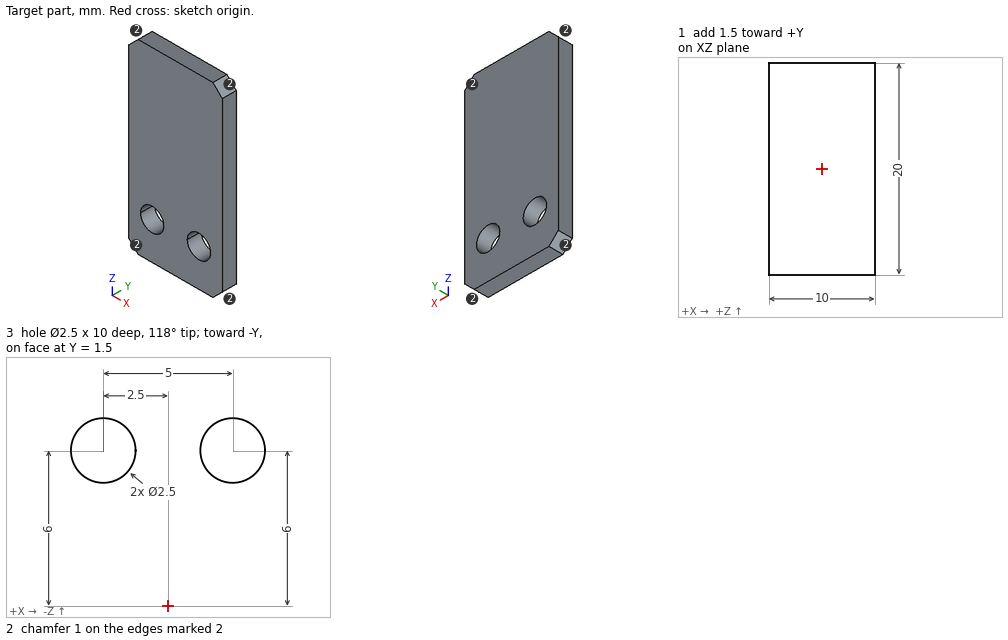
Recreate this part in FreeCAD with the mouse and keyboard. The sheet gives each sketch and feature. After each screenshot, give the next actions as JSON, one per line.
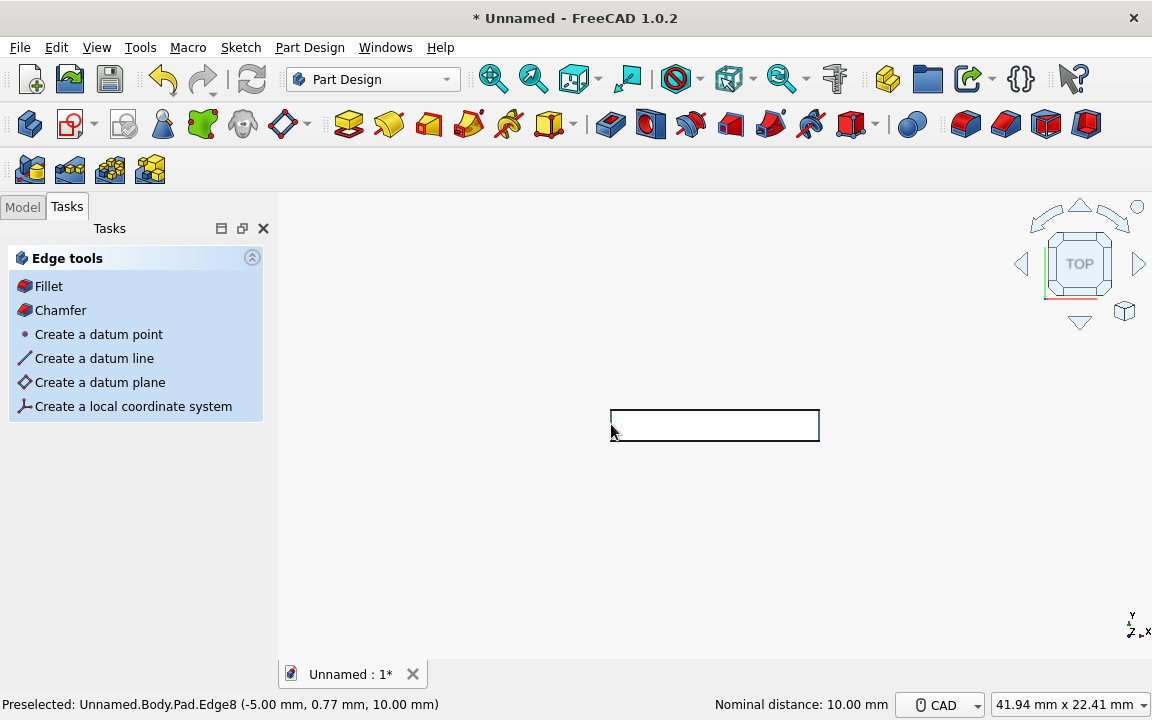
{"action": "key", "text": "1"}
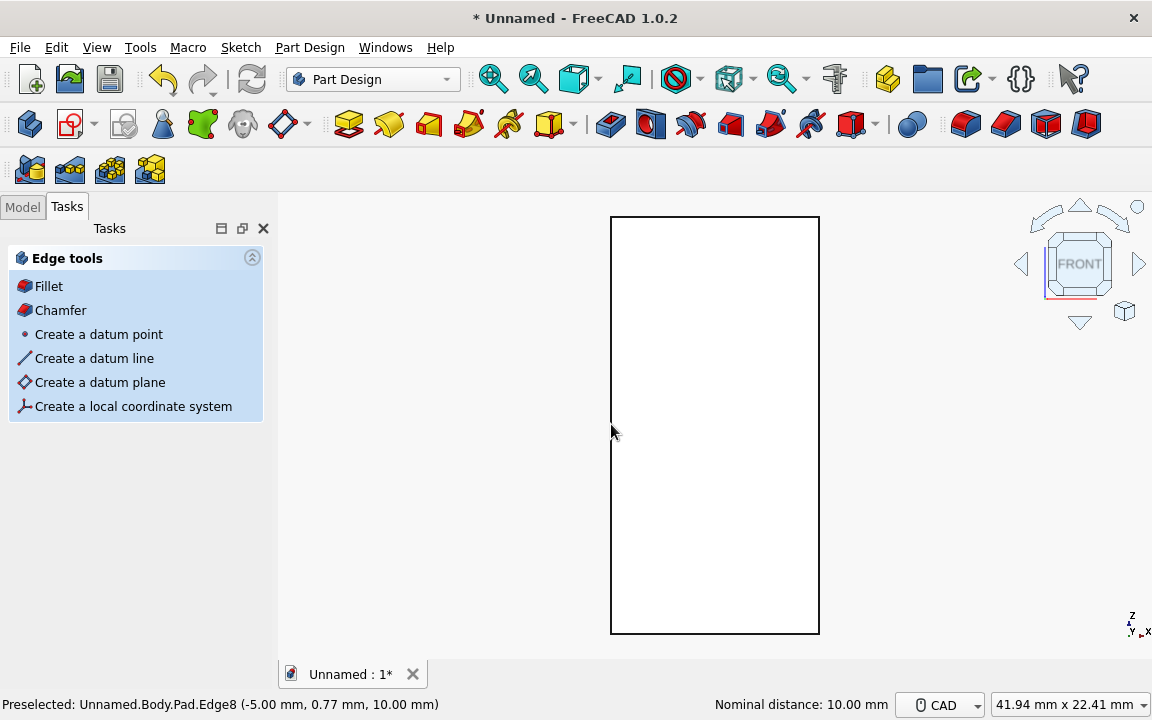
{"action": "key", "text": "3"}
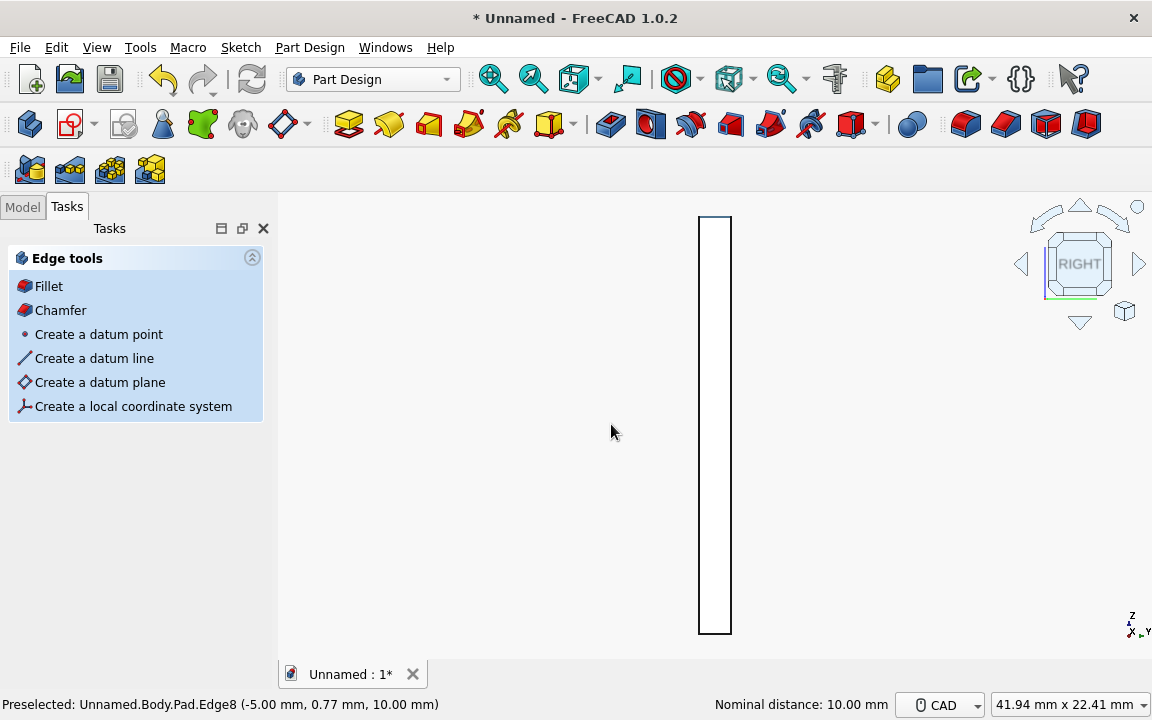
{"action": "key", "text": "5"}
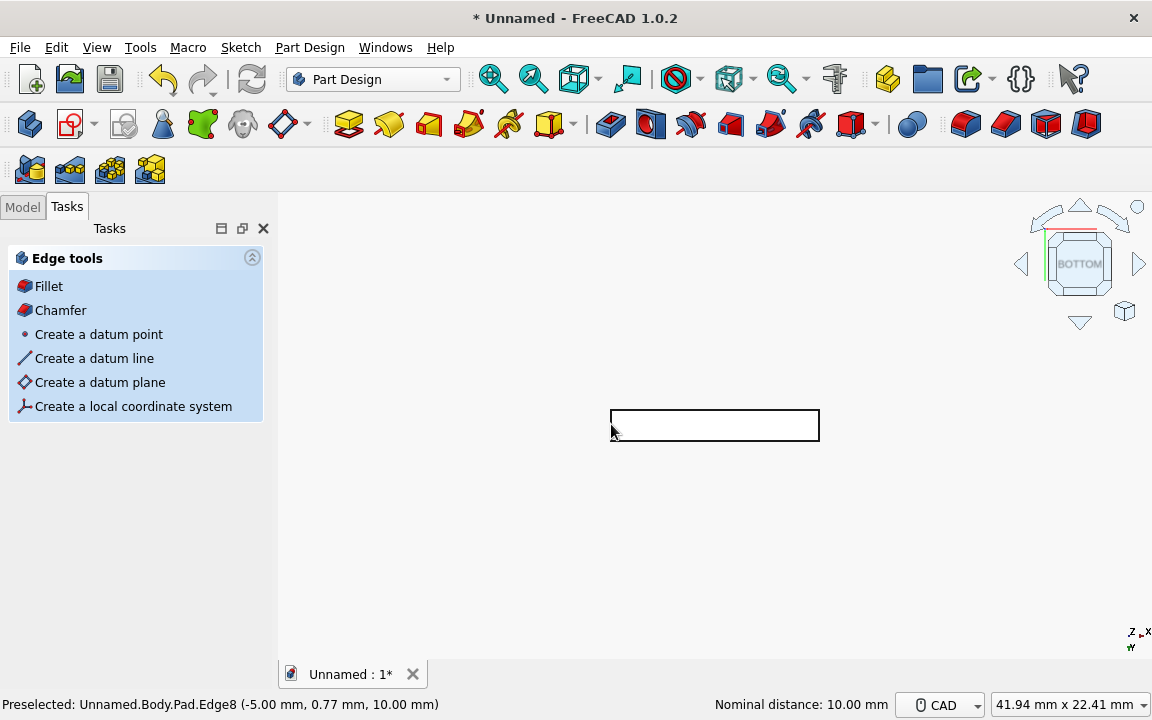
{"action": "left_click", "coordinate": [494, 80]}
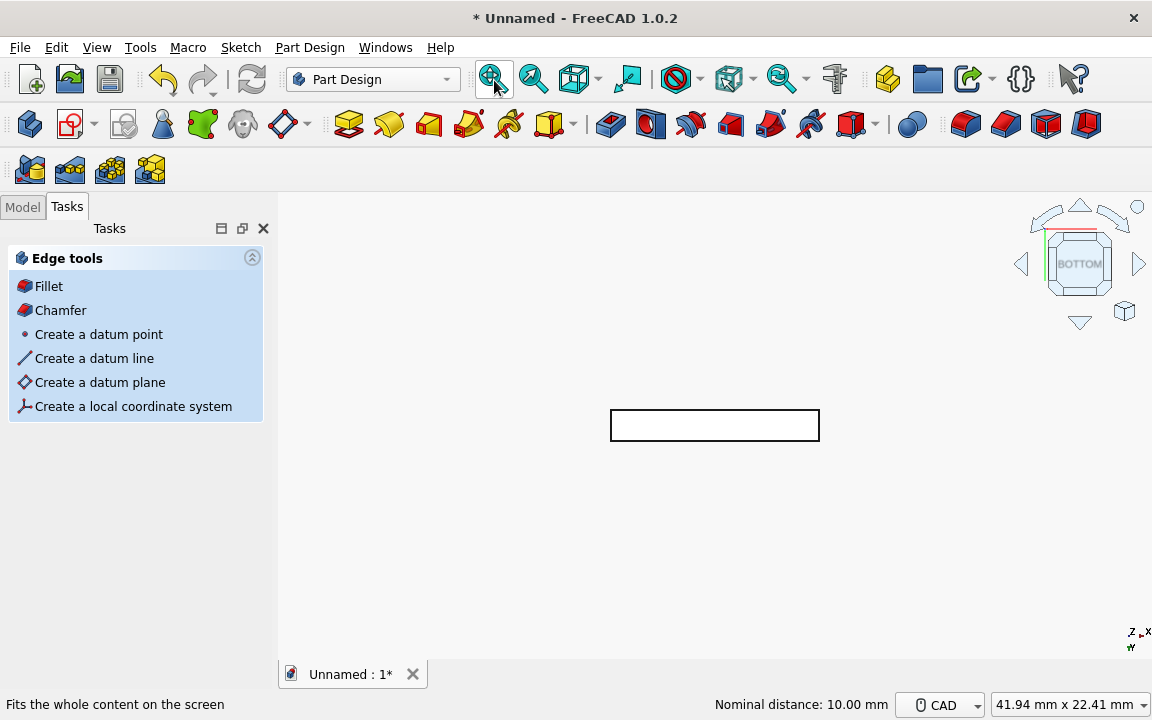
{"action": "left_click", "coordinate": [611, 424], "text": "ctrl"}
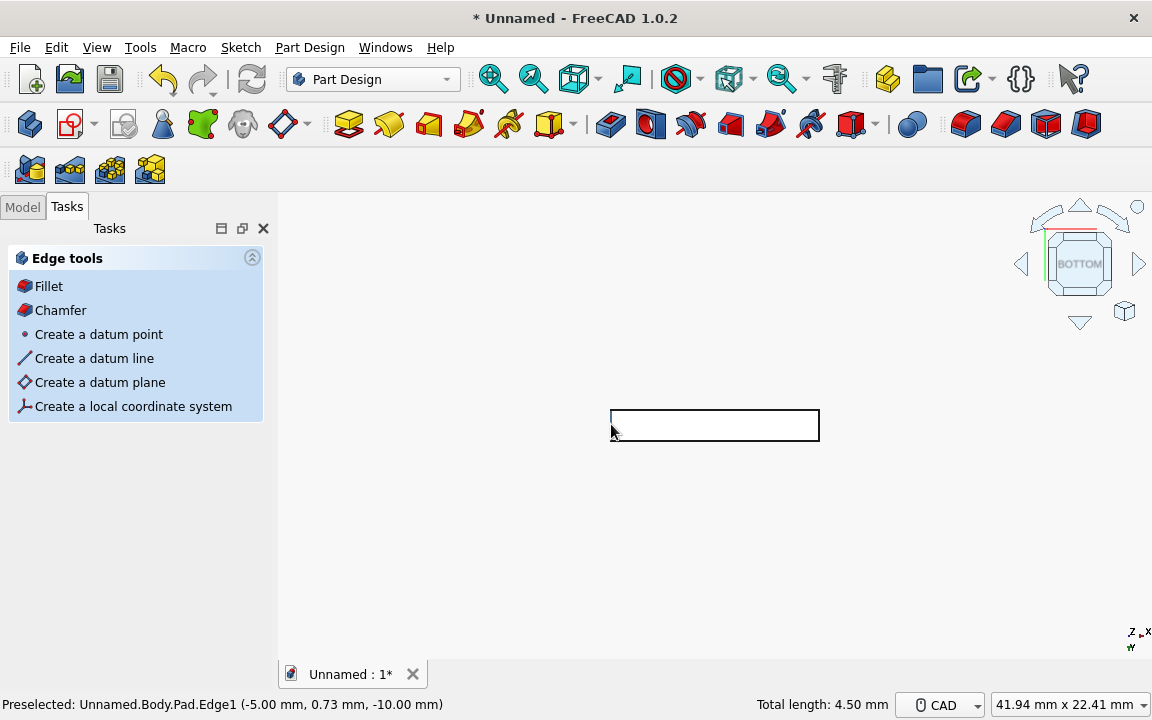
{"action": "left_click", "coordinate": [819, 424], "text": "ctrl"}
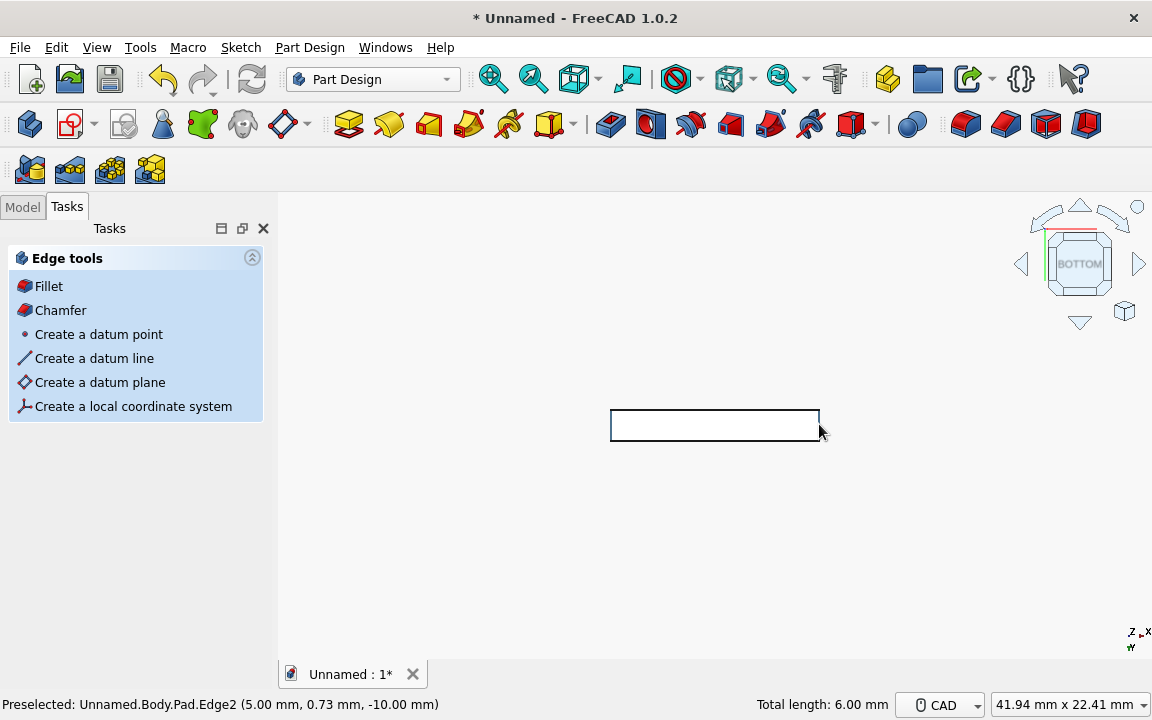
{"action": "left_click", "coordinate": [1006, 124]}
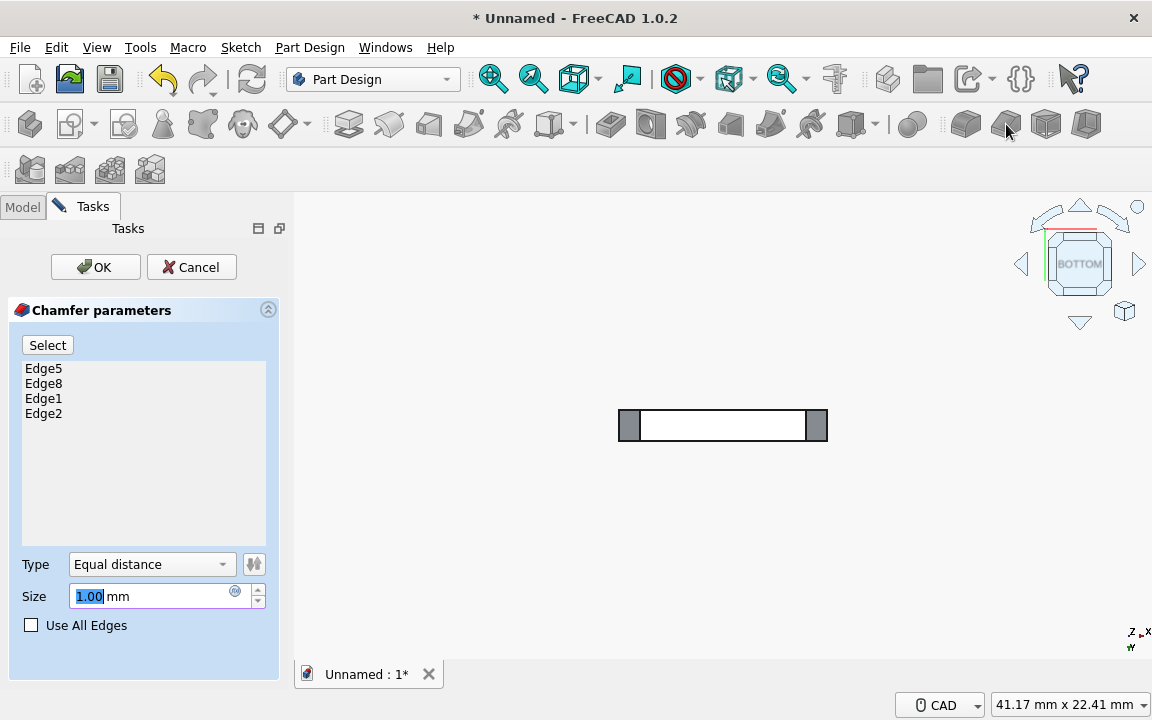
{"action": "type", "text": "1"}
{"action": "key", "text": "Tab"}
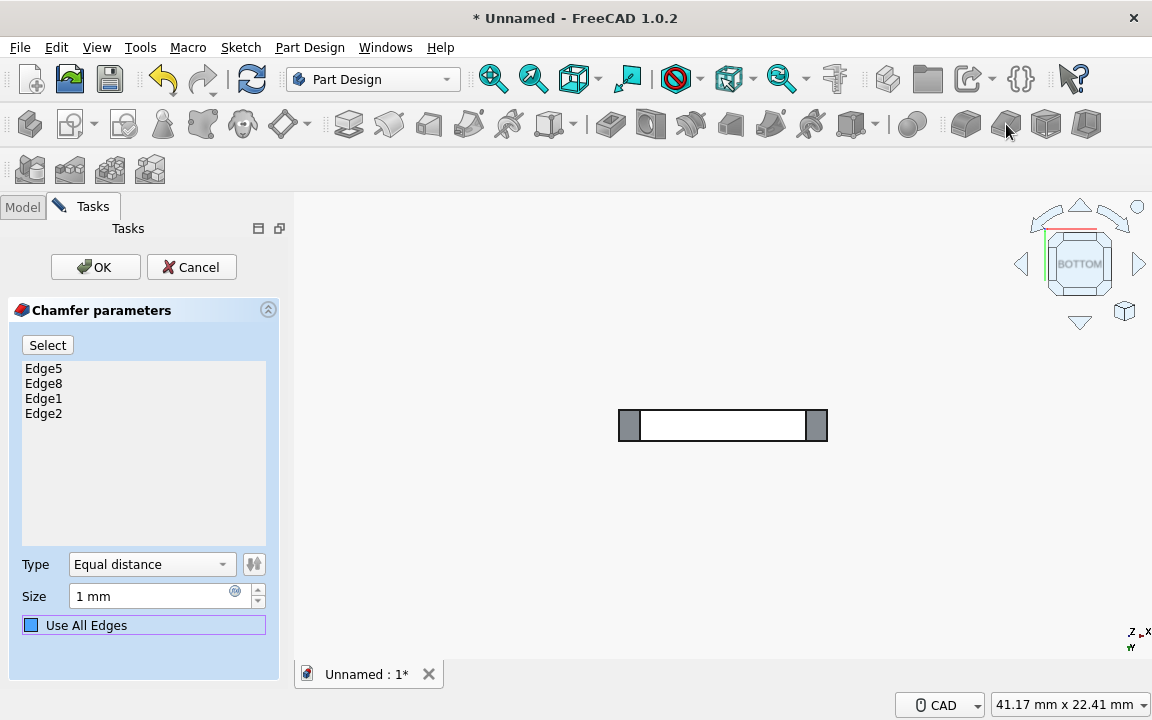
{"action": "left_click", "coordinate": [96, 267]}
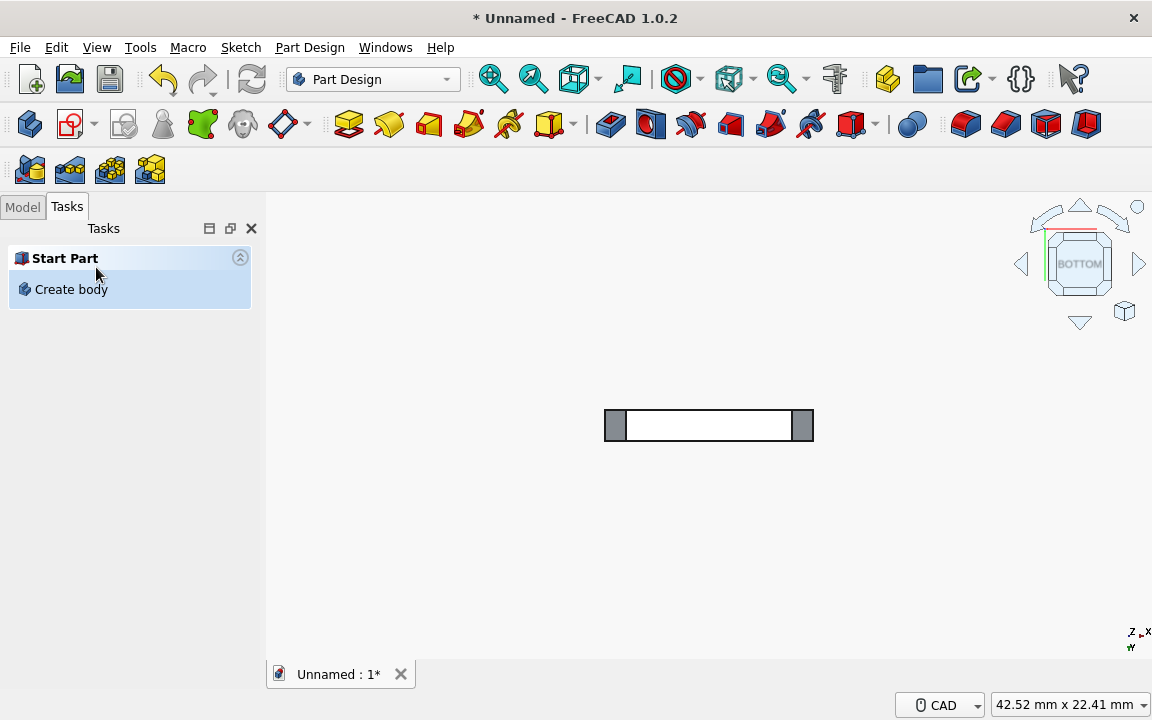
{"action": "key", "text": "v f"}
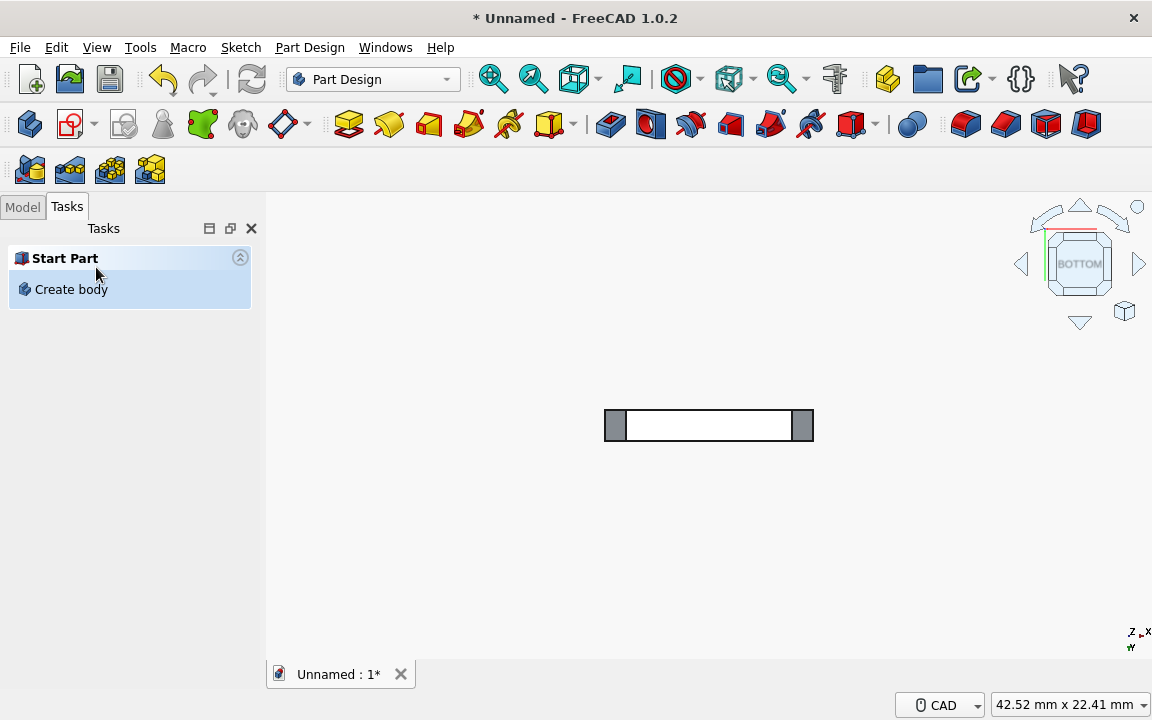
{"action": "key", "text": "4"}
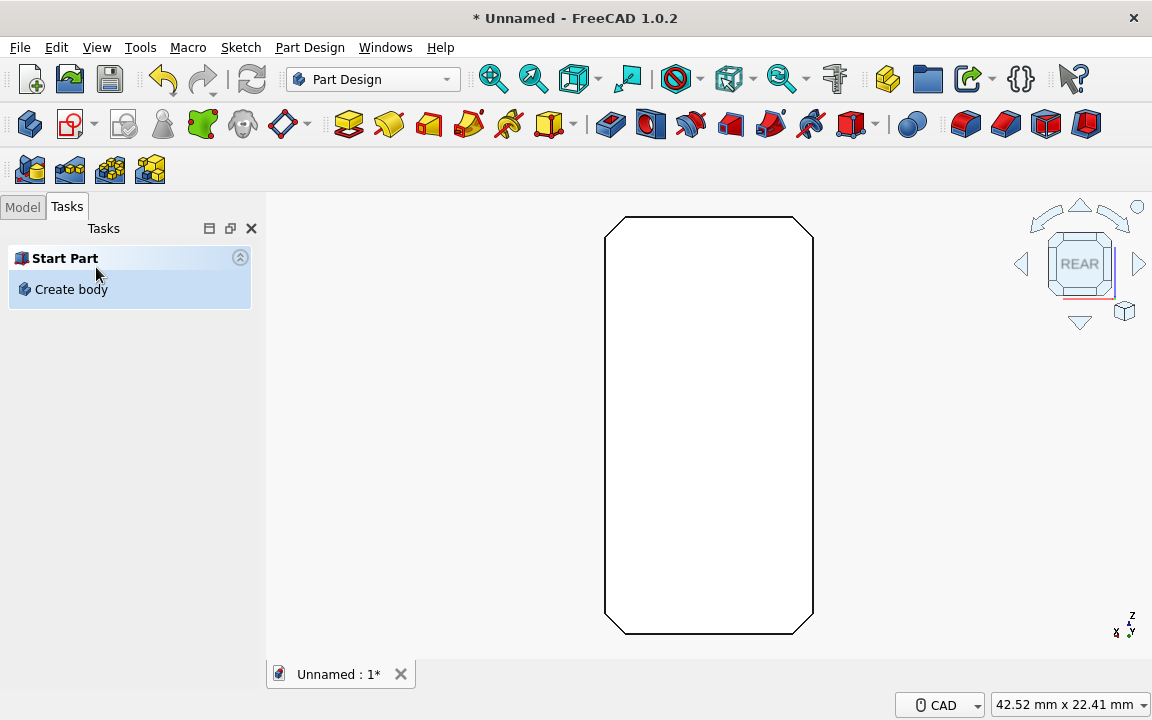
{"action": "left_click", "coordinate": [709, 365]}